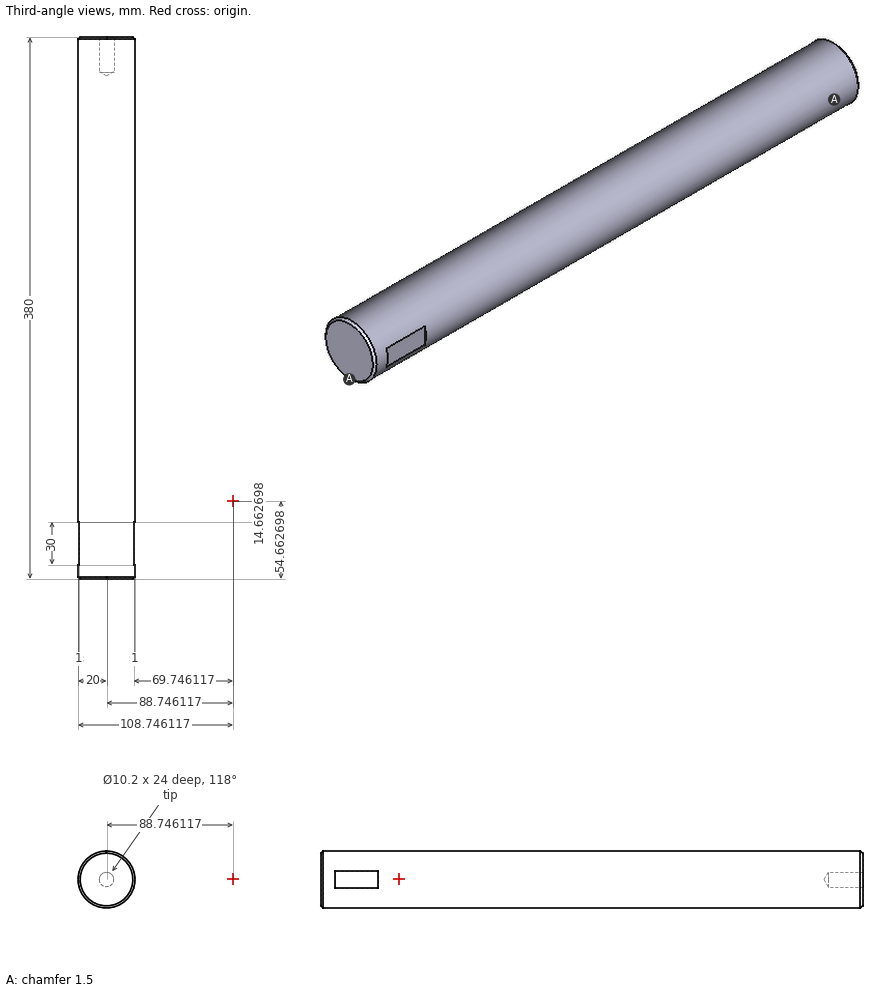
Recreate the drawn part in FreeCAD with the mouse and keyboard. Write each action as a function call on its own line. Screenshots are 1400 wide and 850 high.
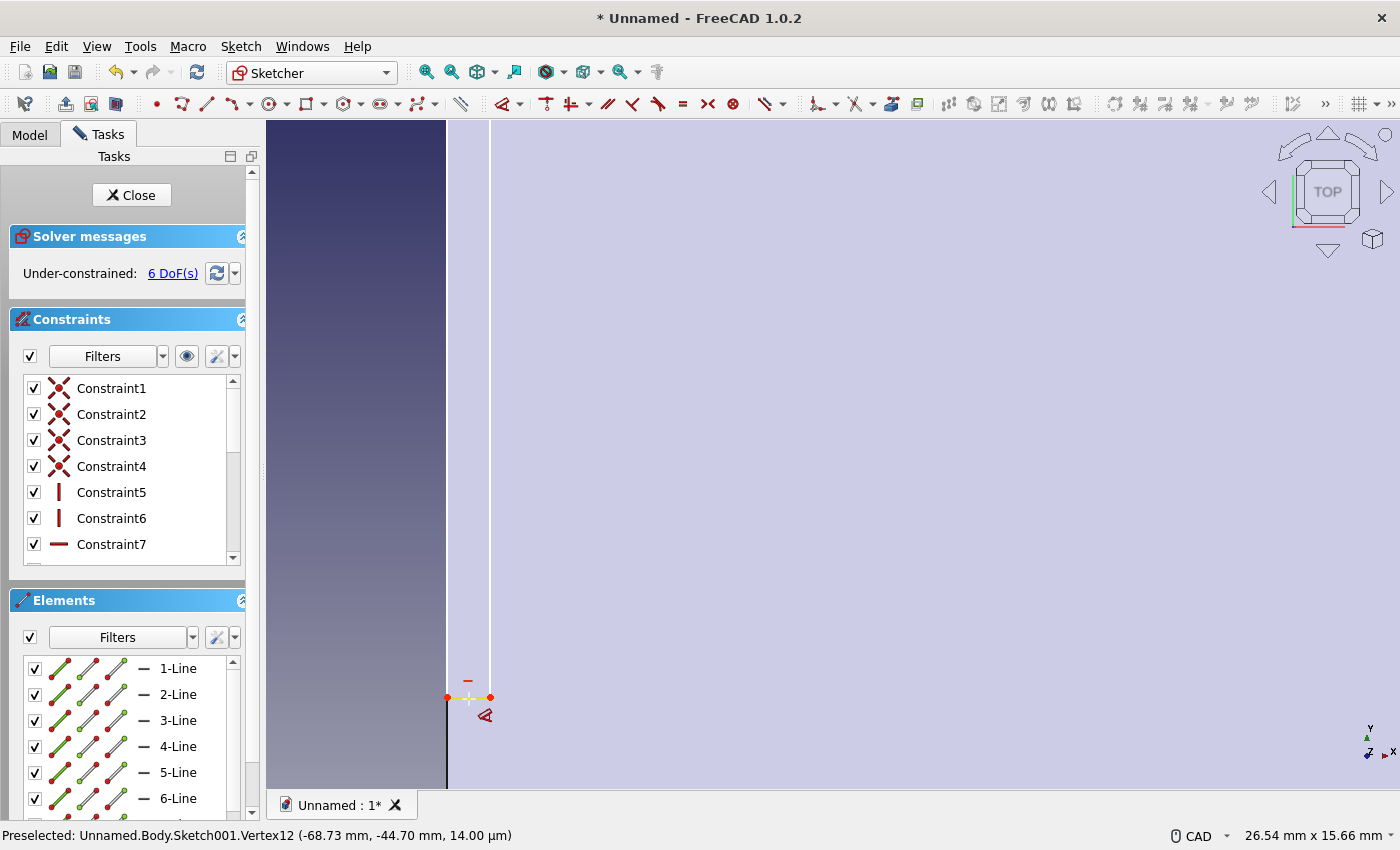
click(469, 698)
click(469, 732)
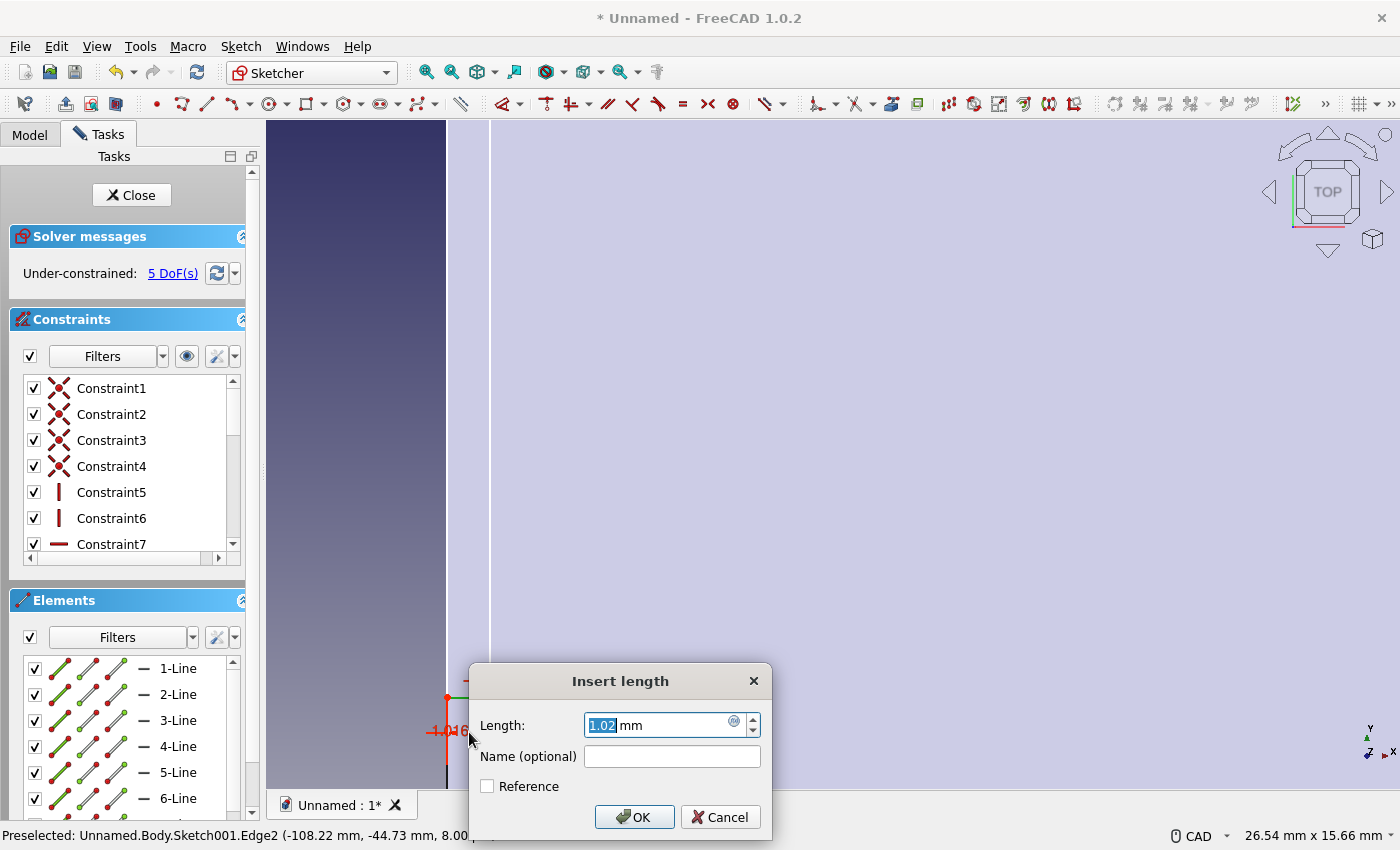
text(1)
key(Return)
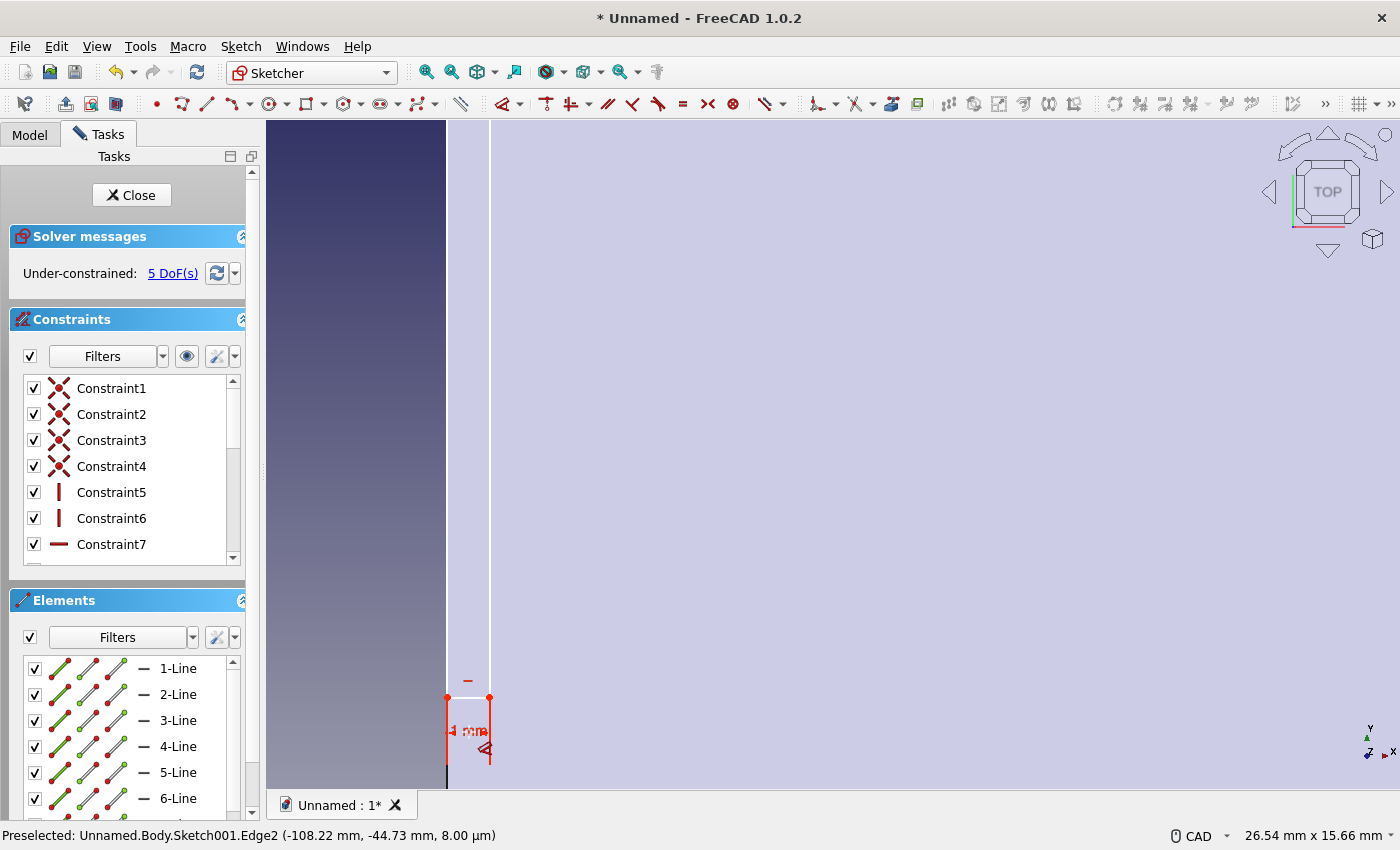
click(447, 313)
click(413, 423)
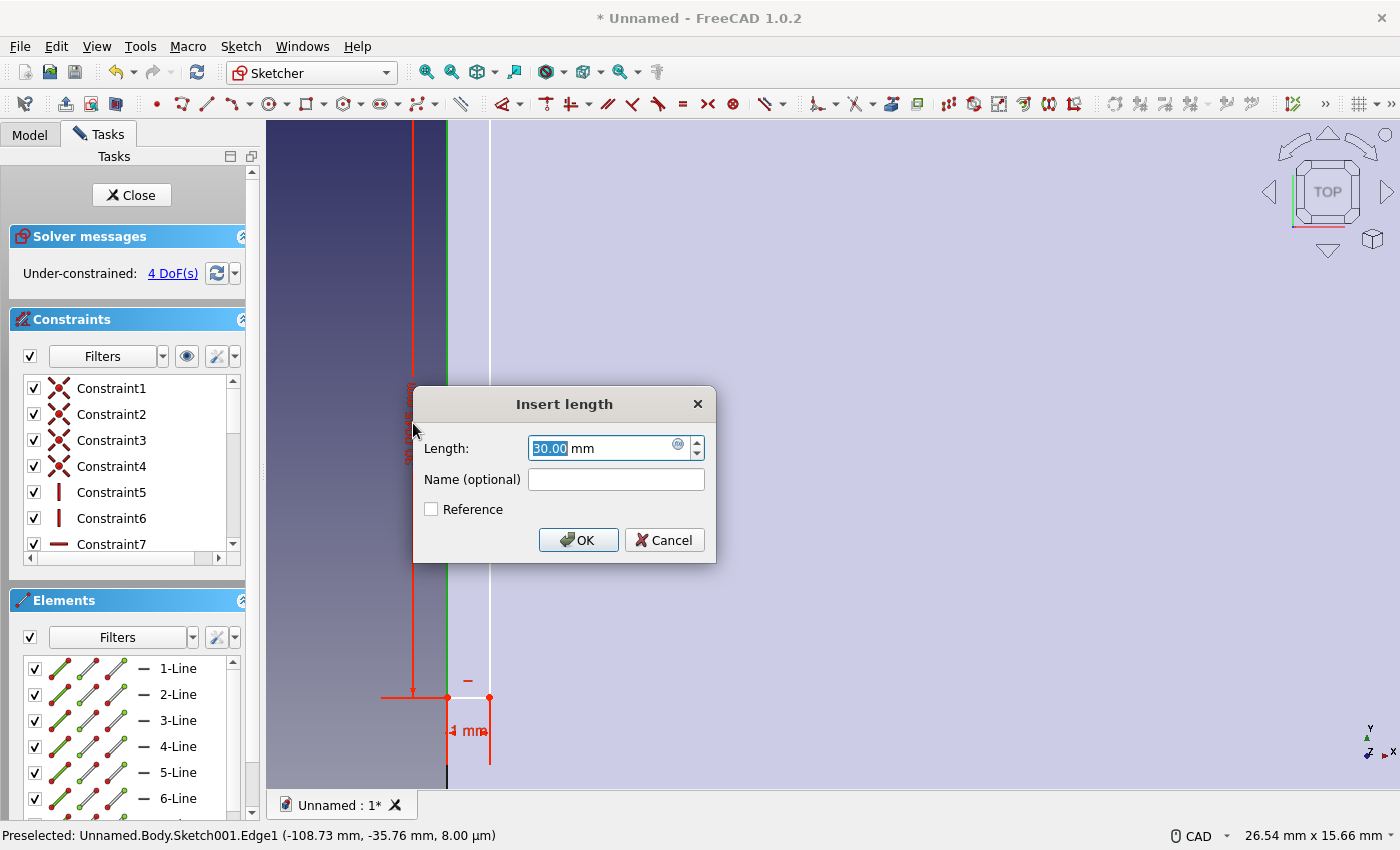
text(30)
key(Return)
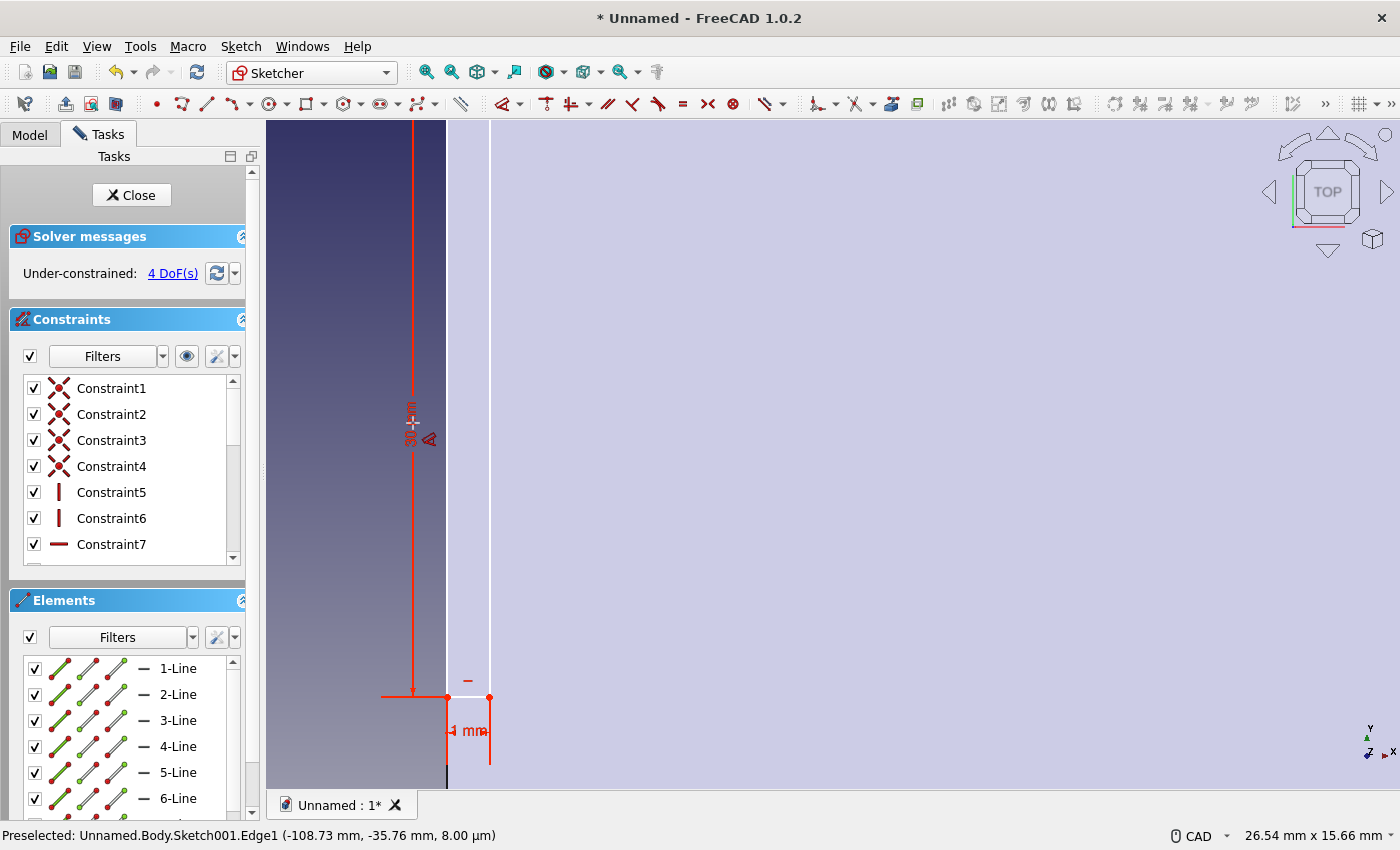
scroll(452, 688, down, 5)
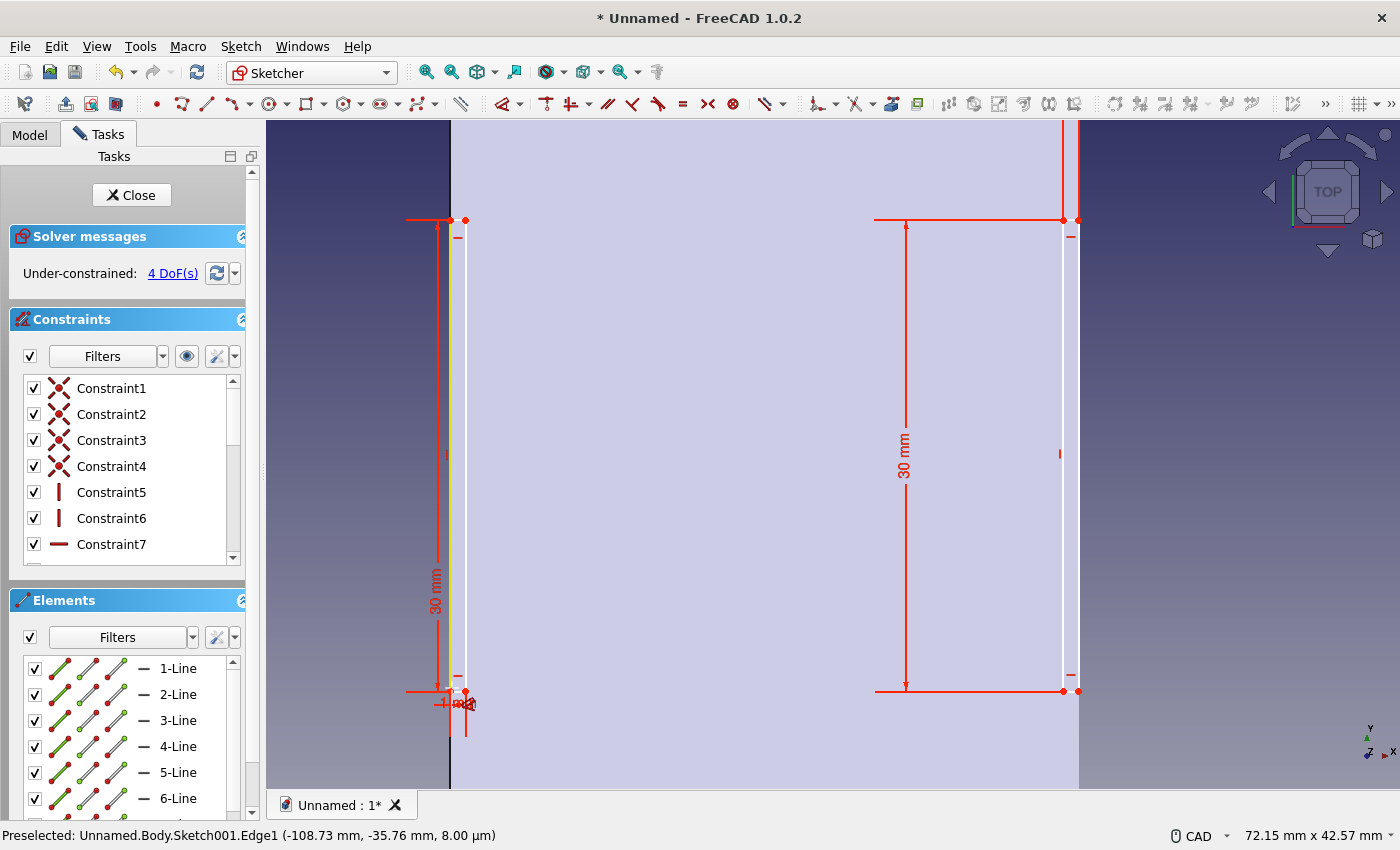
click(450, 220)
click(416, 184)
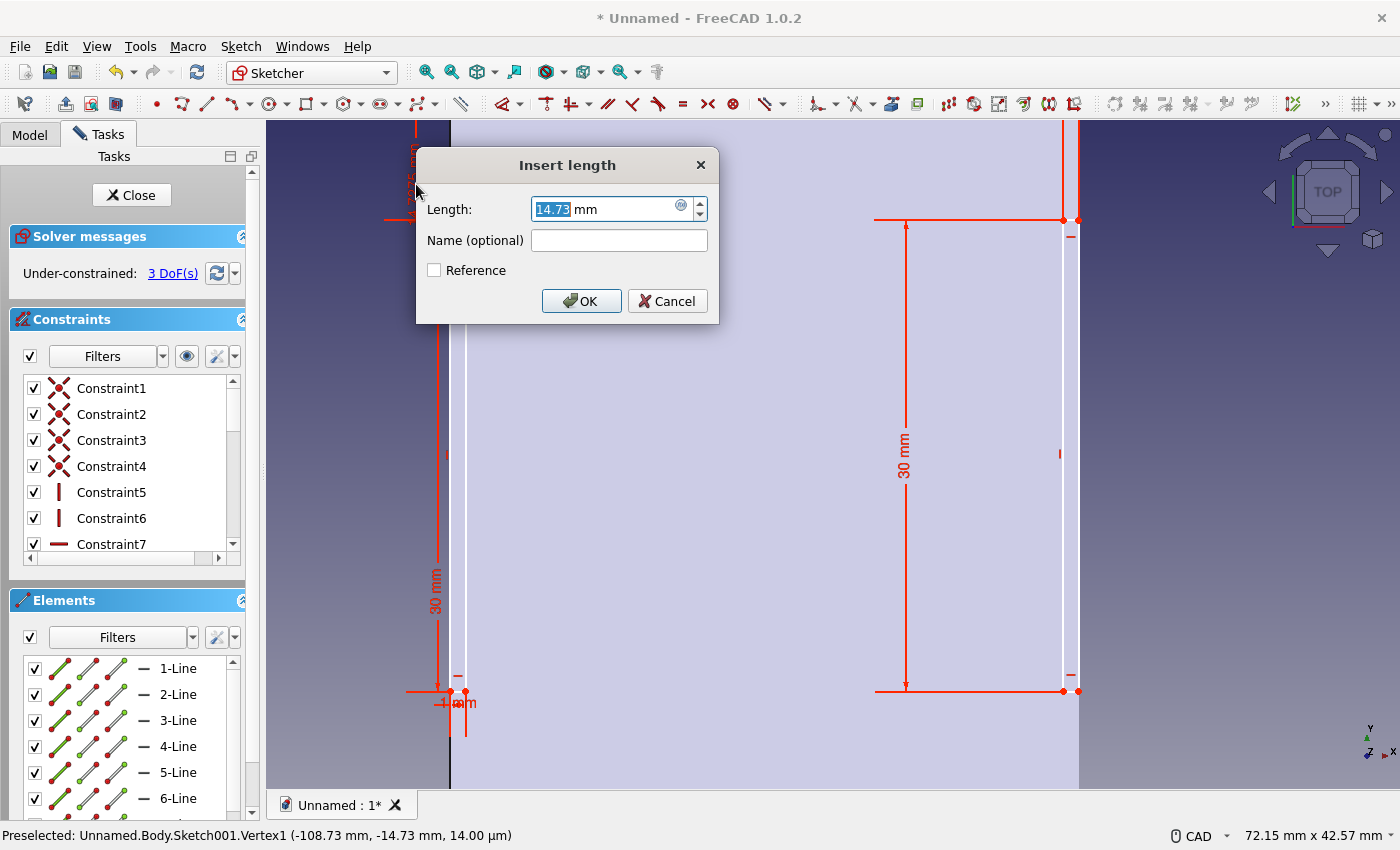
text(14.662698)
key(Return)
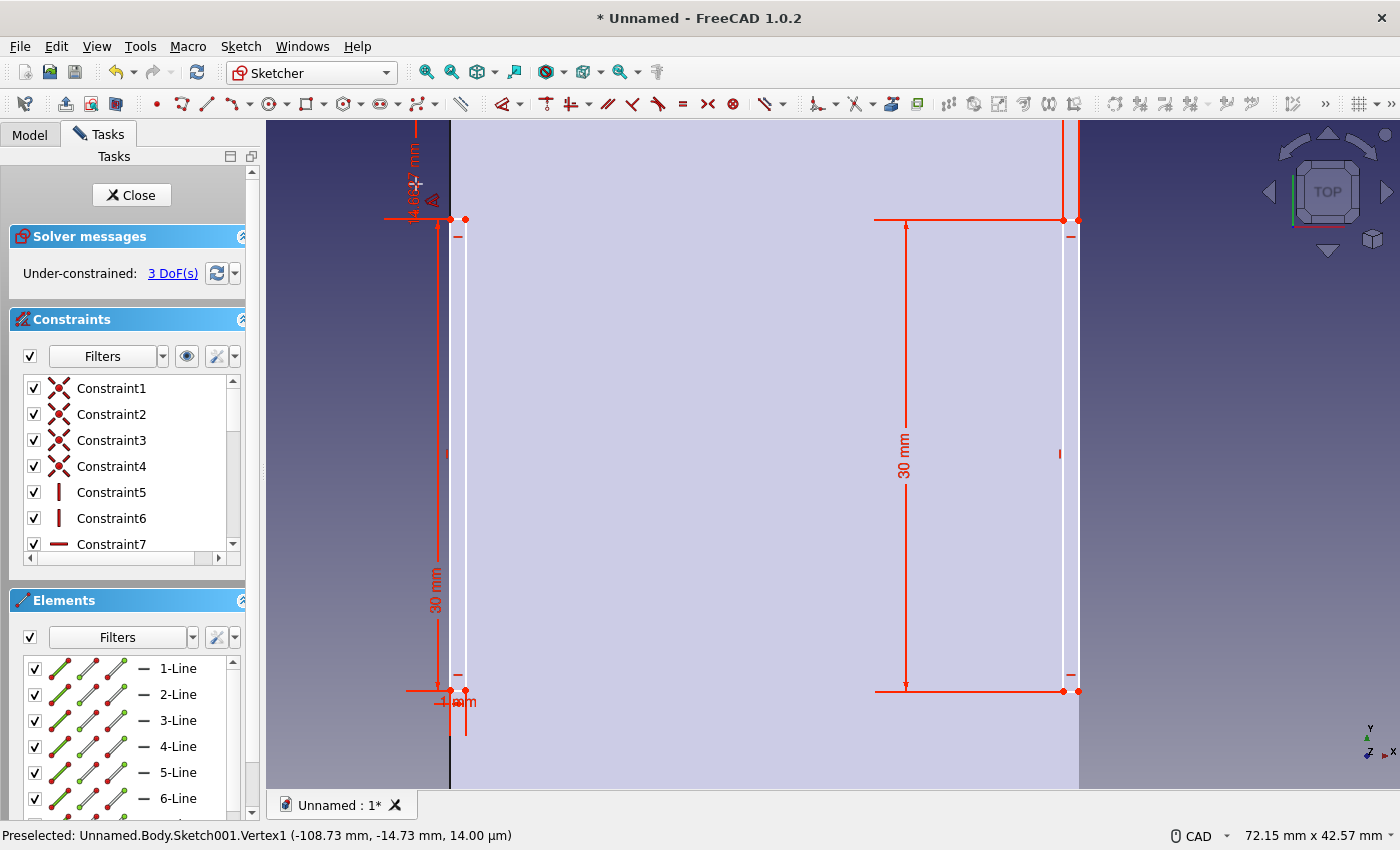
click(1063, 220)
click(1149, 254)